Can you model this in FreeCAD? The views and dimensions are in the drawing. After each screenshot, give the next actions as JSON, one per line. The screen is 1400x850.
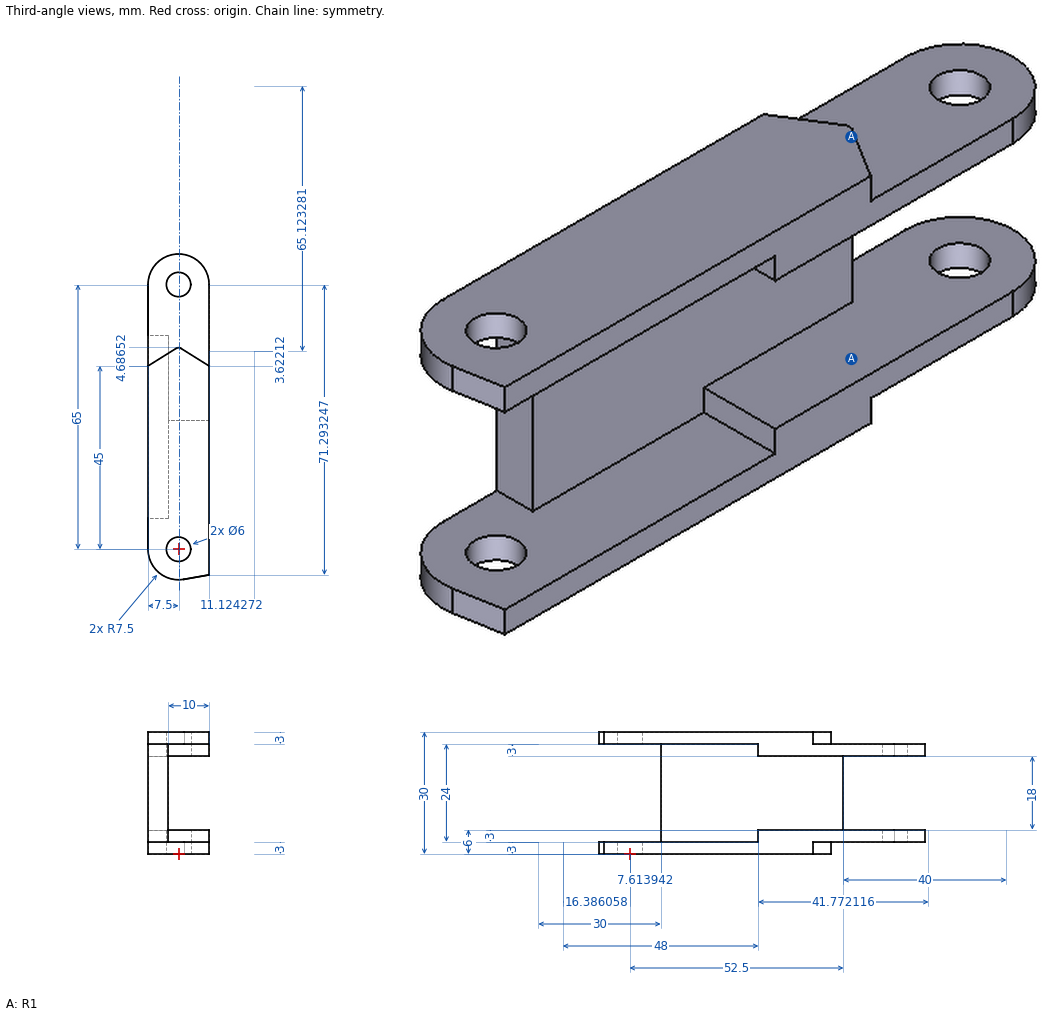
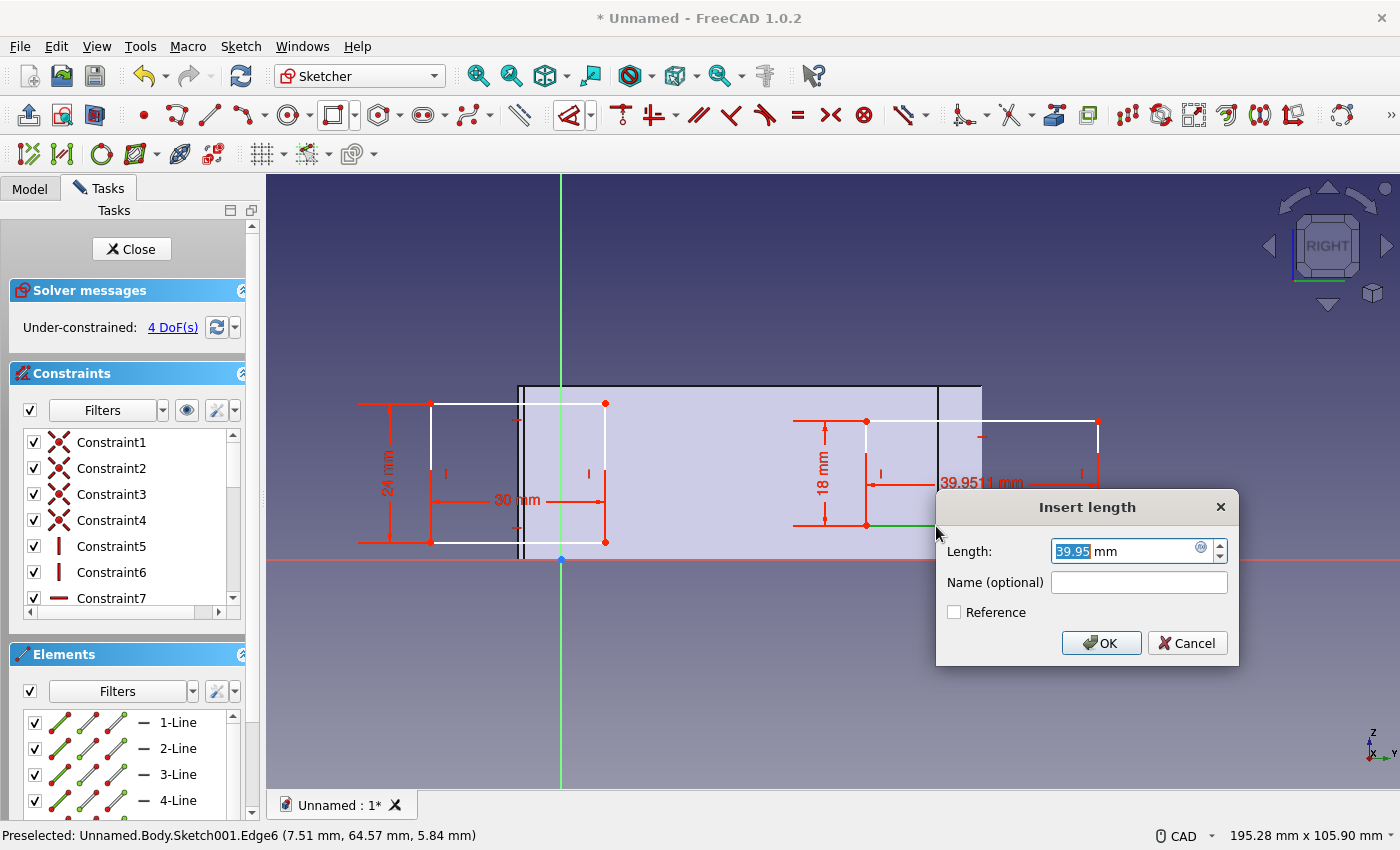
{"action": "type", "text": "40"}
{"action": "key", "text": "Return"}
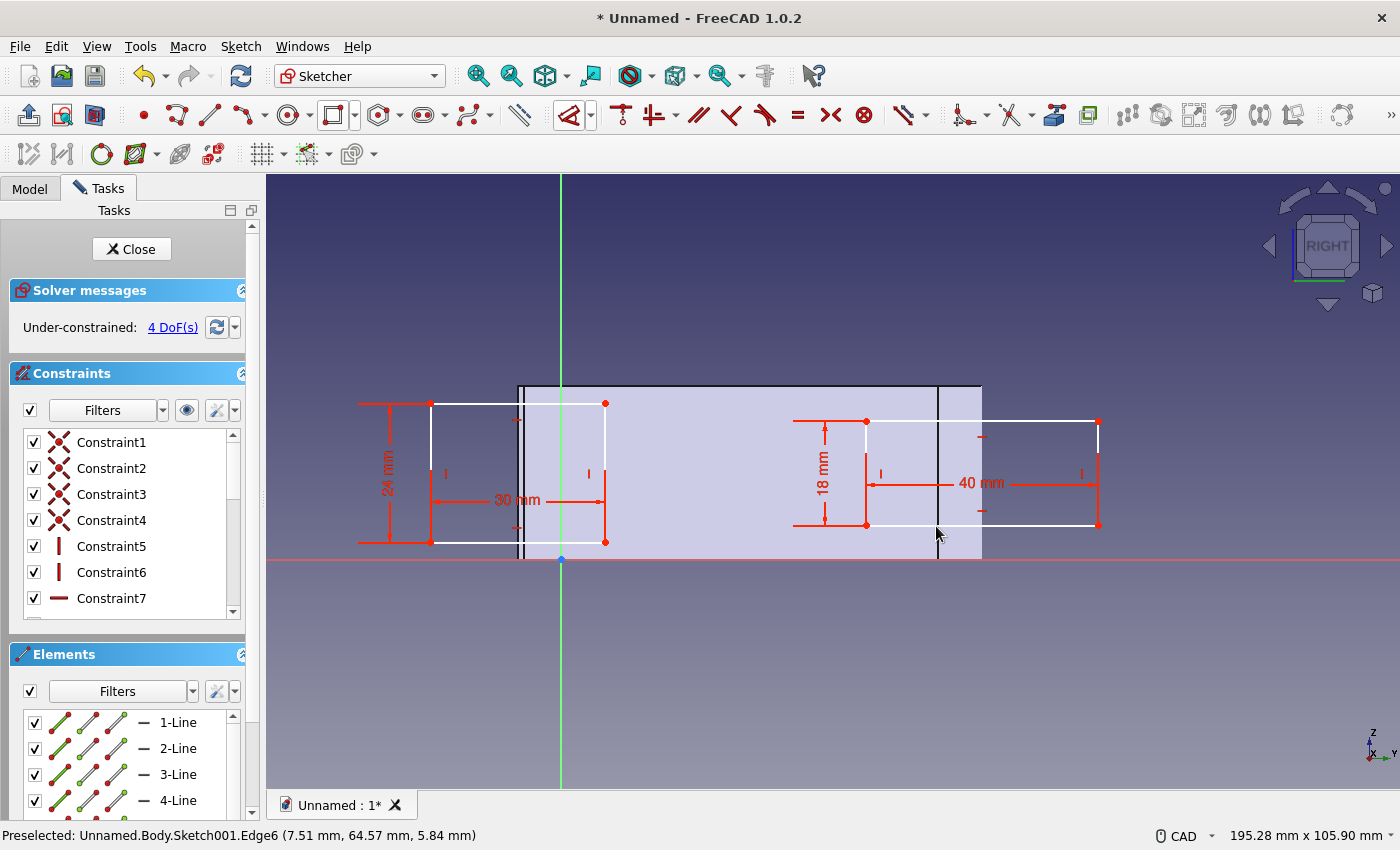
{"action": "scroll", "coordinate": [431, 543], "scroll_direction": "up", "scroll_amount": 5}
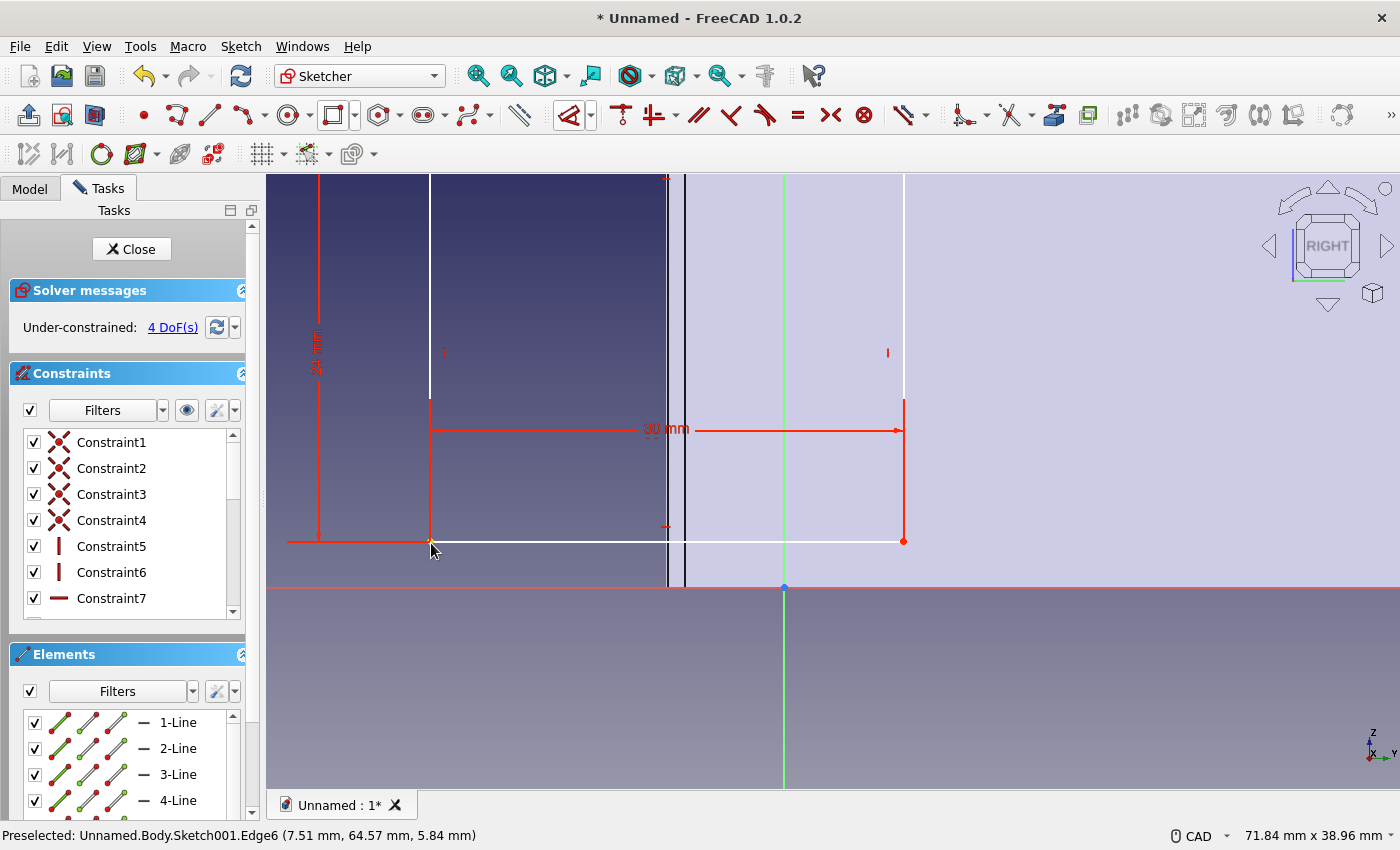
{"action": "left_click", "coordinate": [430, 542]}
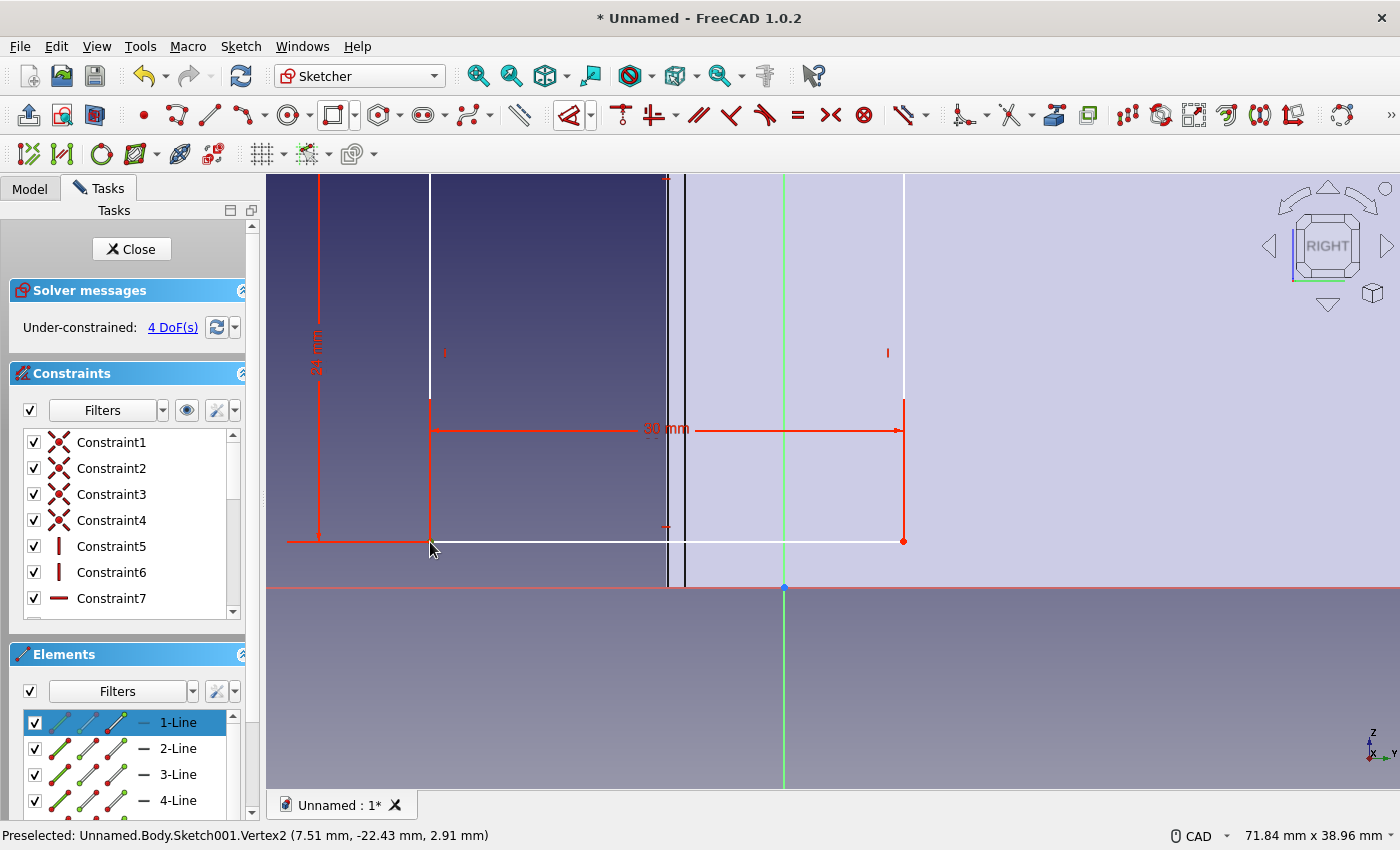
{"action": "key", "text": "i"}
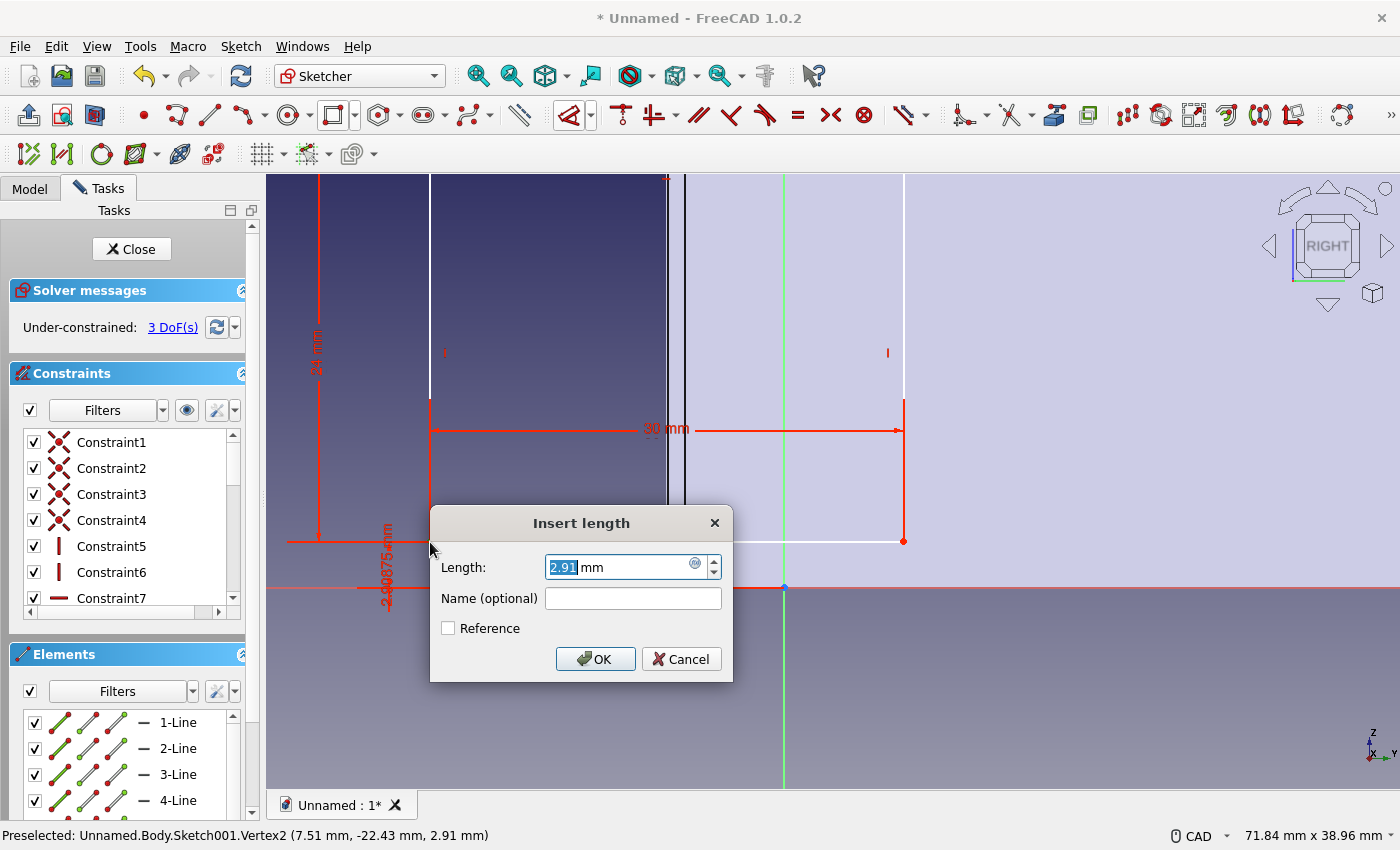
{"action": "type", "text": "3"}
{"action": "key", "text": "Return"}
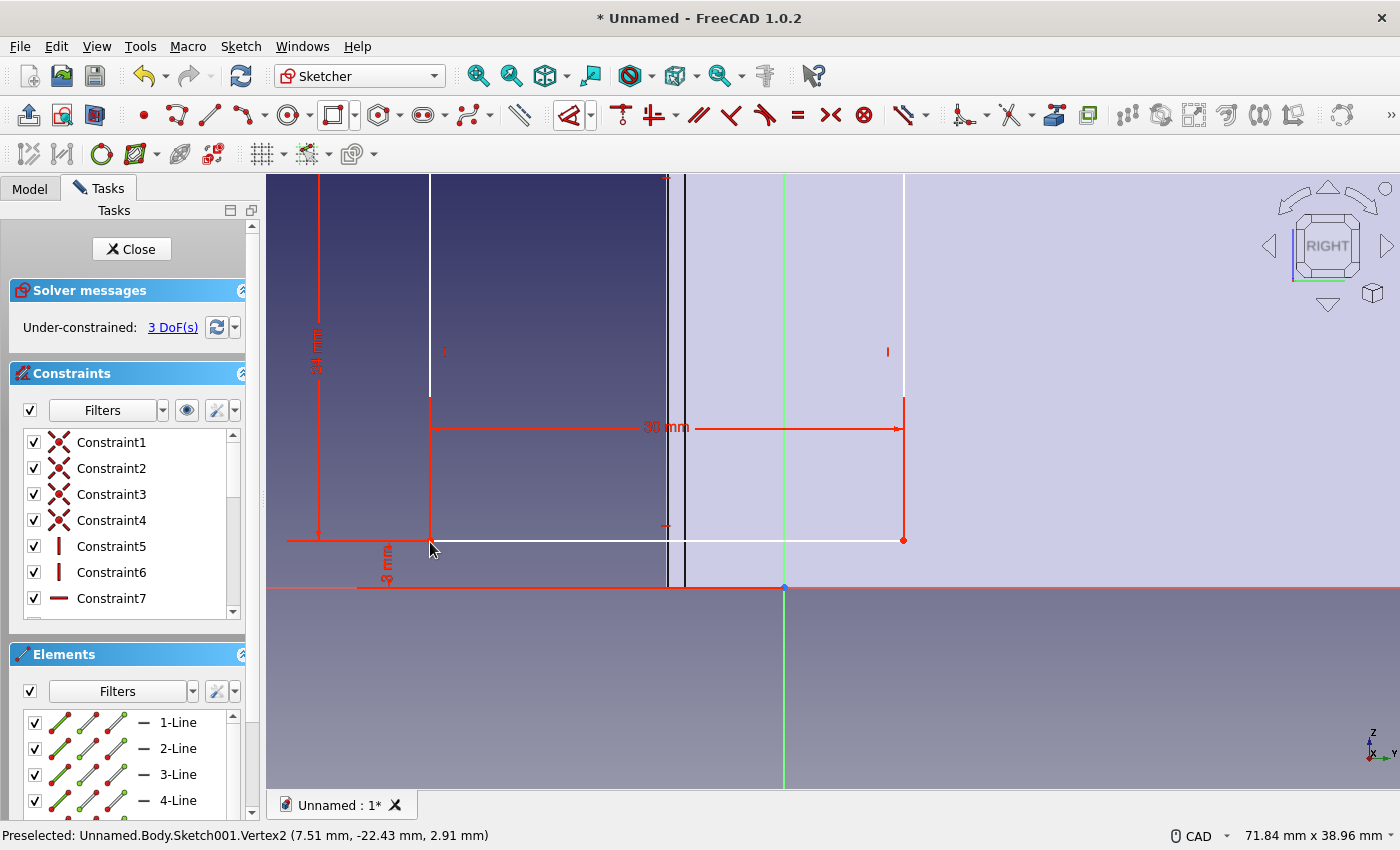
{"action": "scroll", "coordinate": [431, 544], "scroll_direction": "down", "scroll_amount": 5}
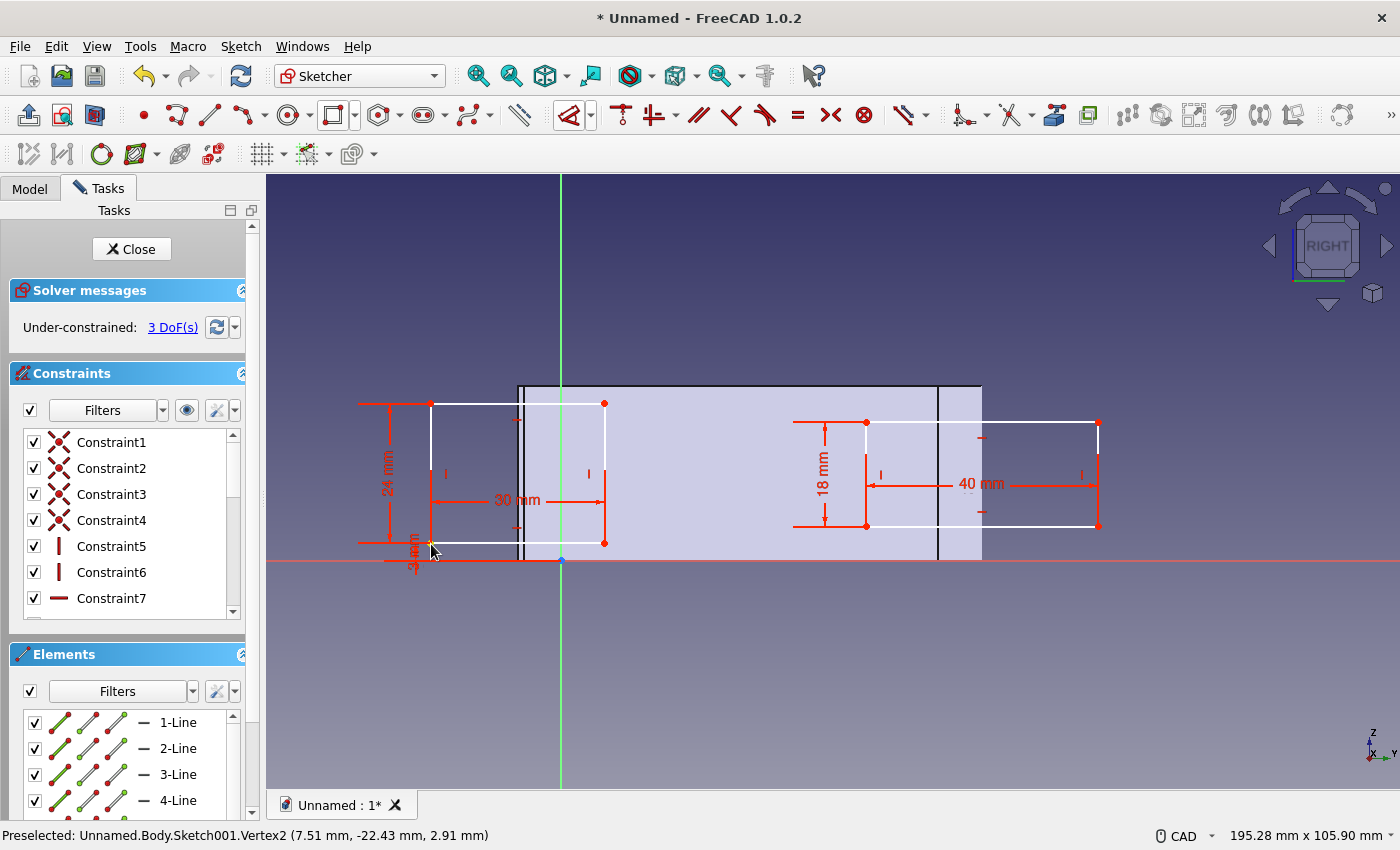
{"action": "left_click", "coordinate": [866, 527]}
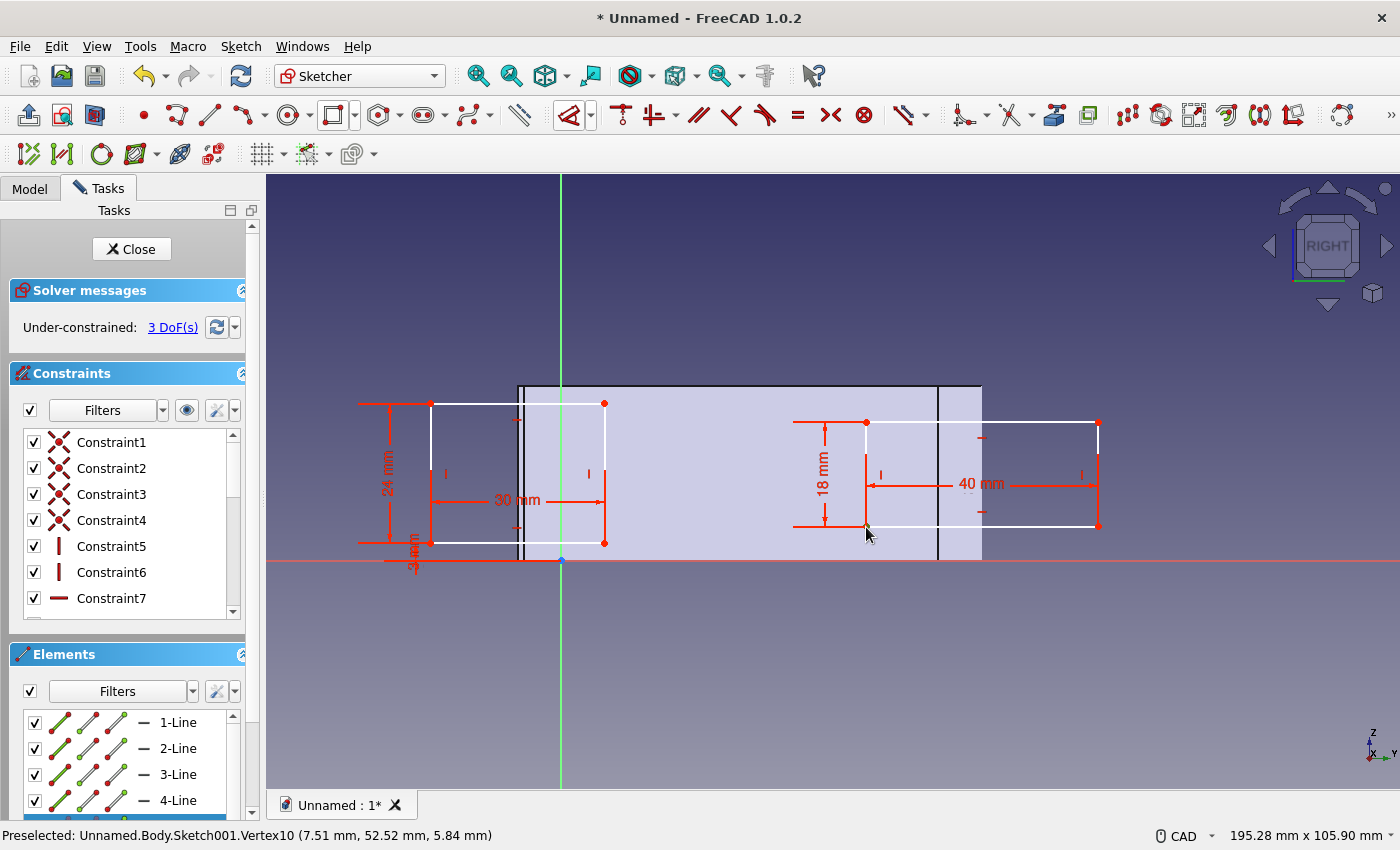
{"action": "key", "text": "i"}